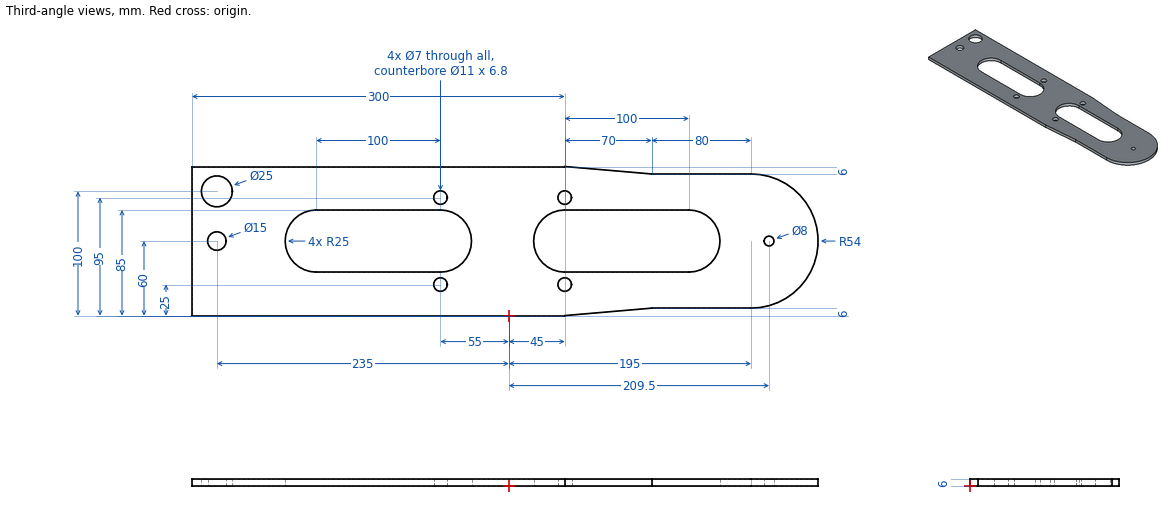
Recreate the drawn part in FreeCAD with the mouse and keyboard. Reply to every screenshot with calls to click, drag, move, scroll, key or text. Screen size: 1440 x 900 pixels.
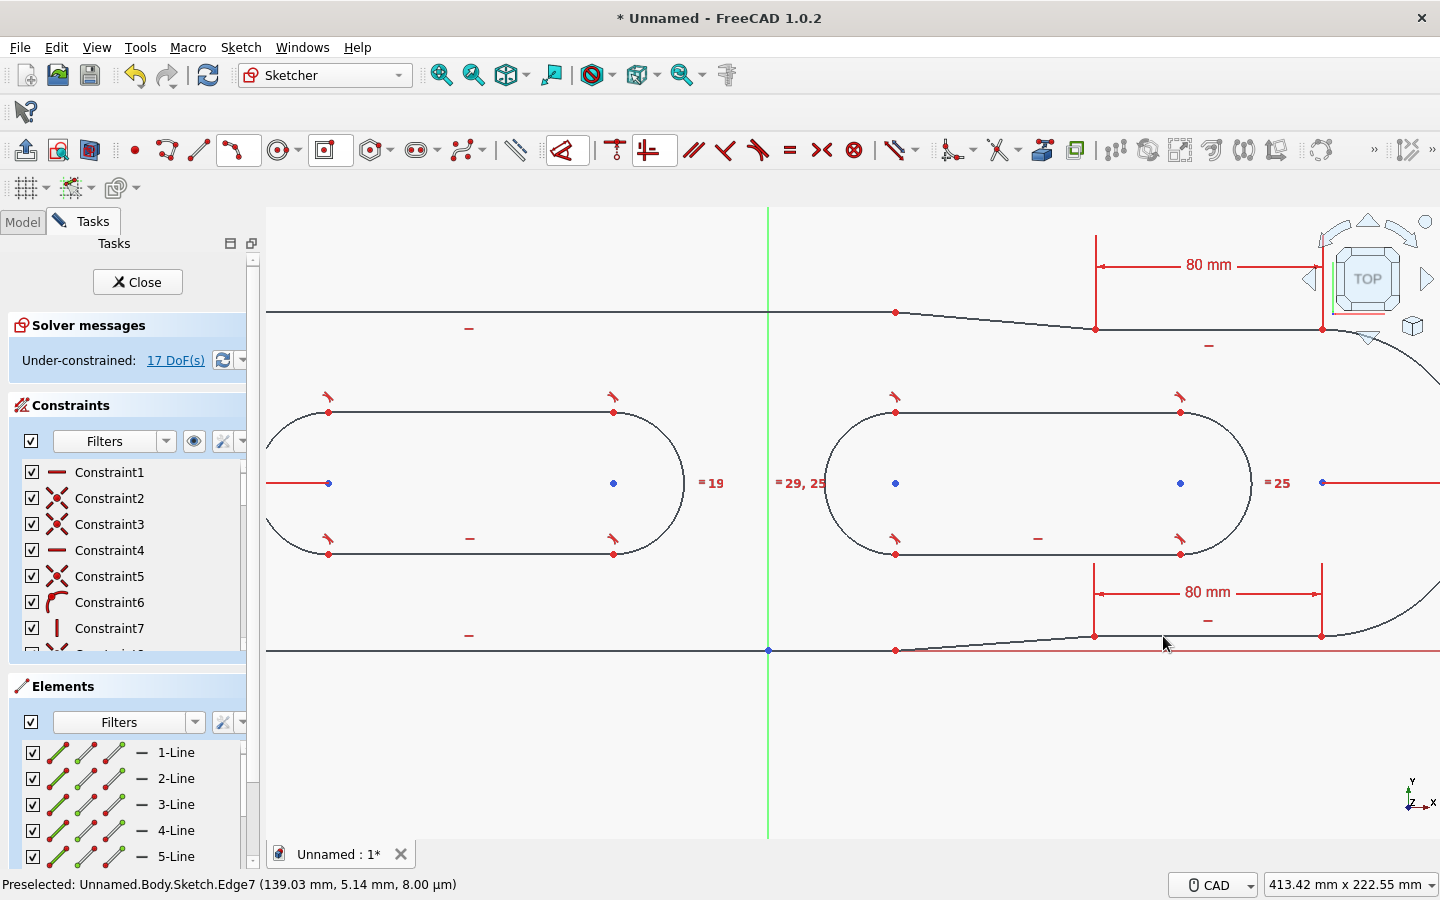
scroll(1094, 636, up, 5)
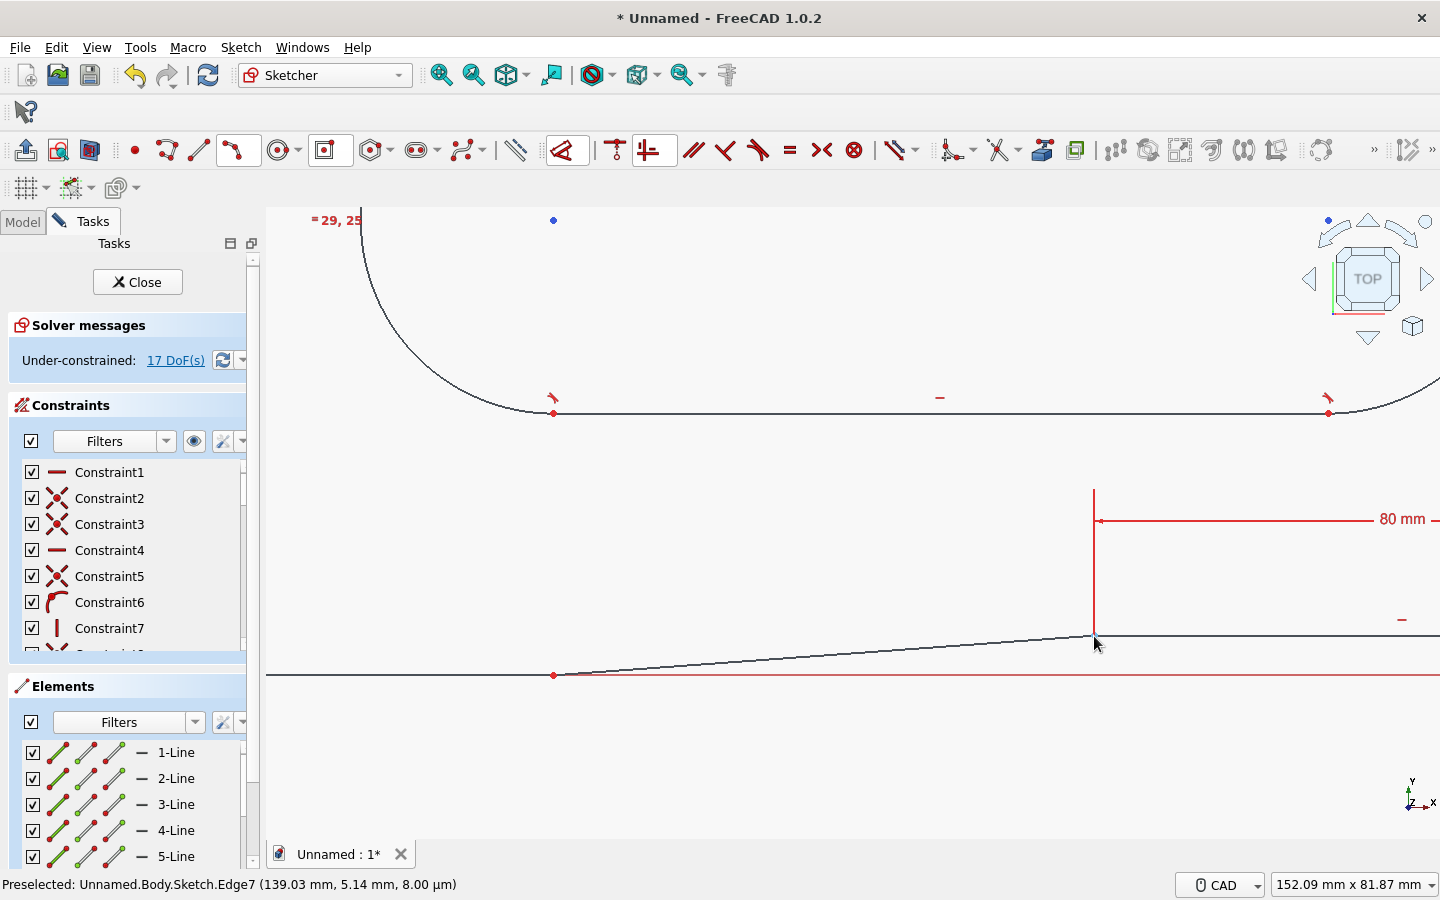
click(1094, 636)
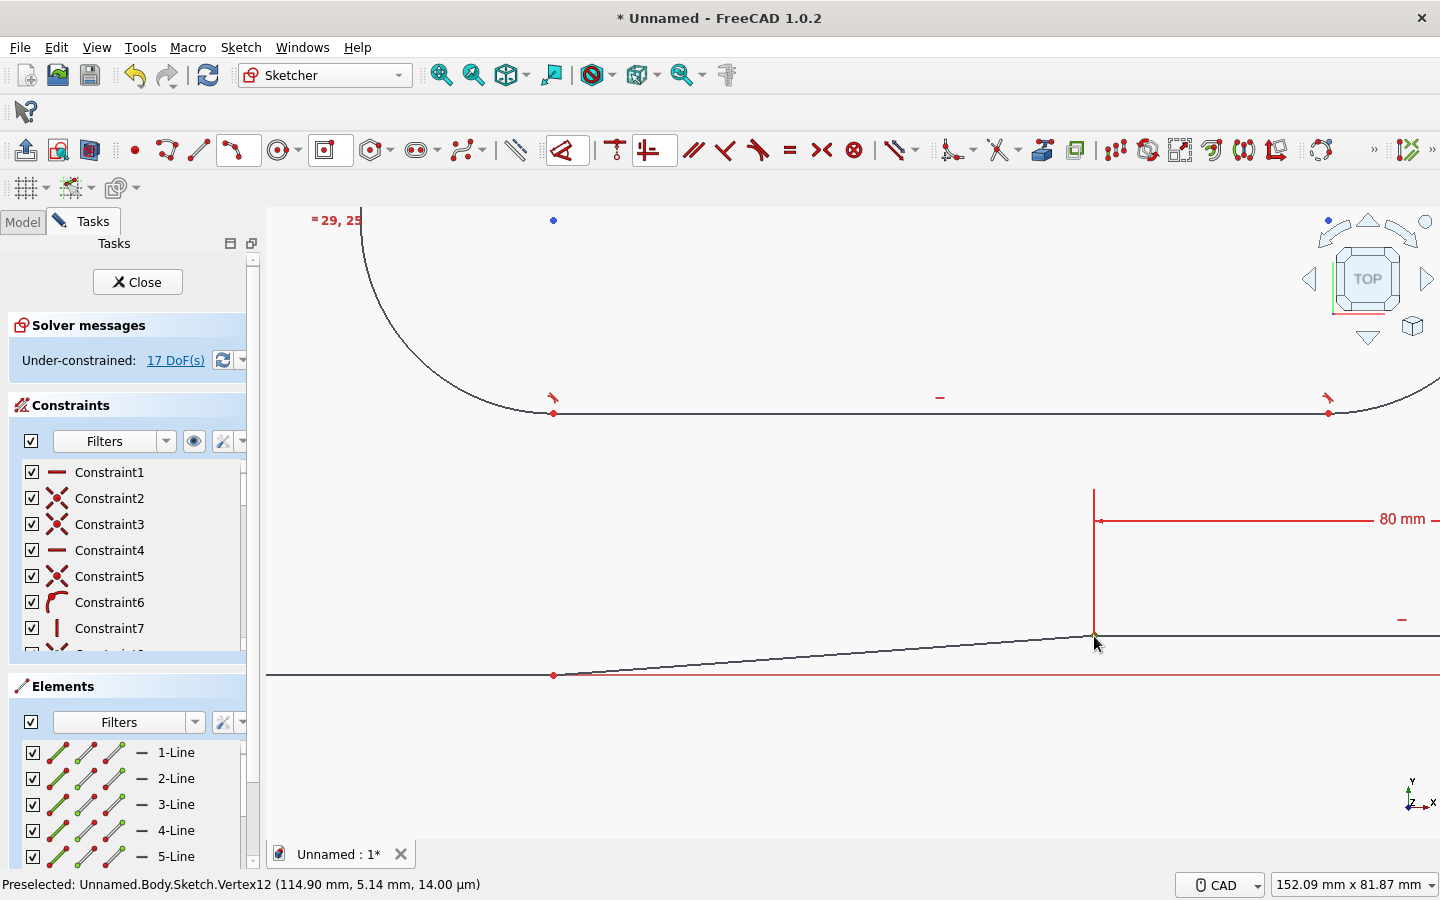
key(i)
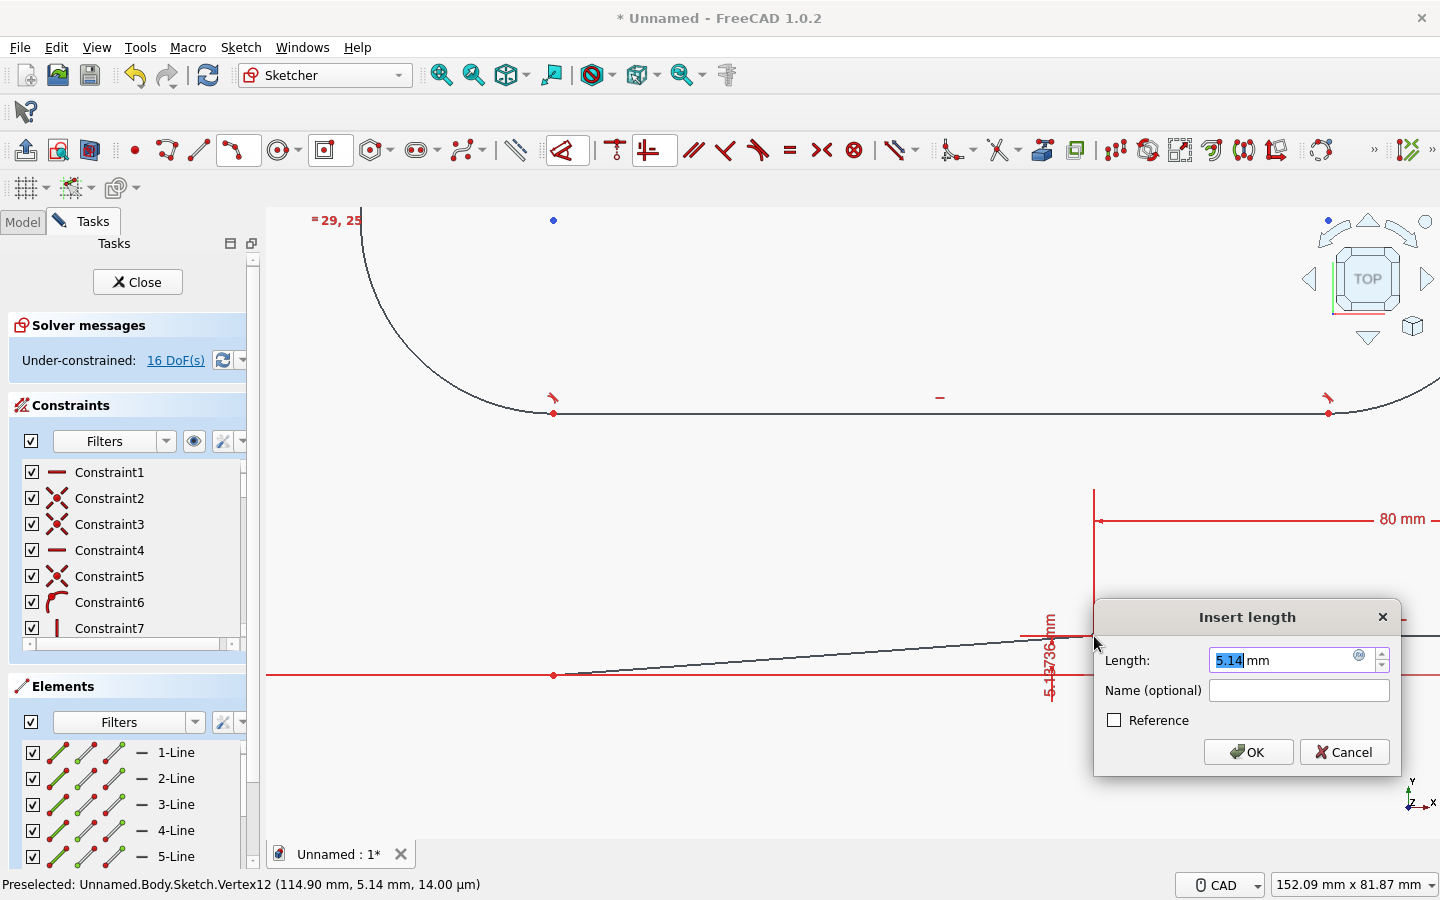
text(6)
key(Return)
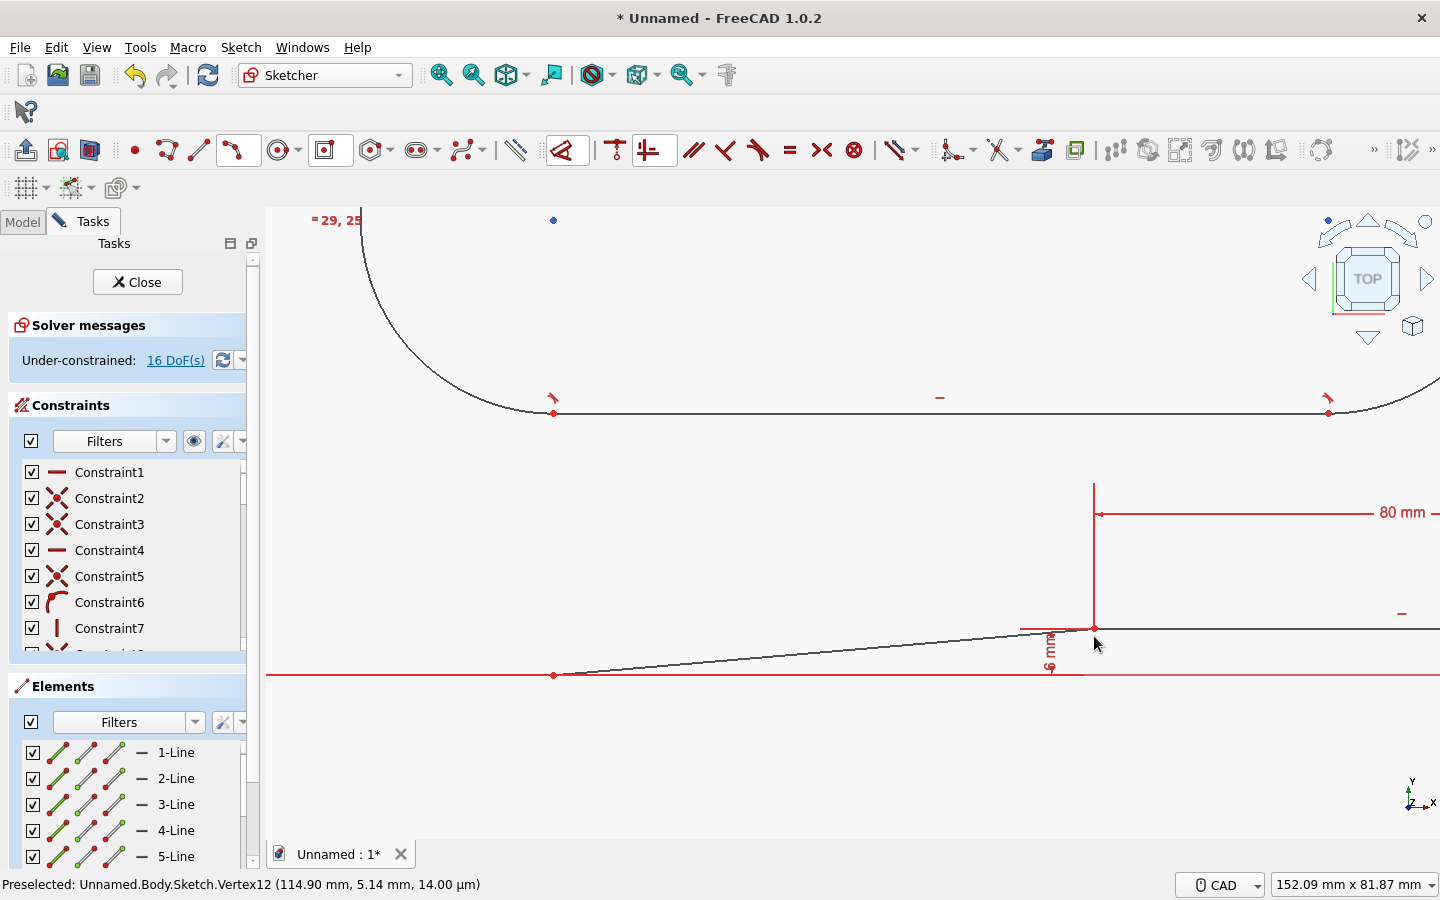
scroll(903, 585, down, 9)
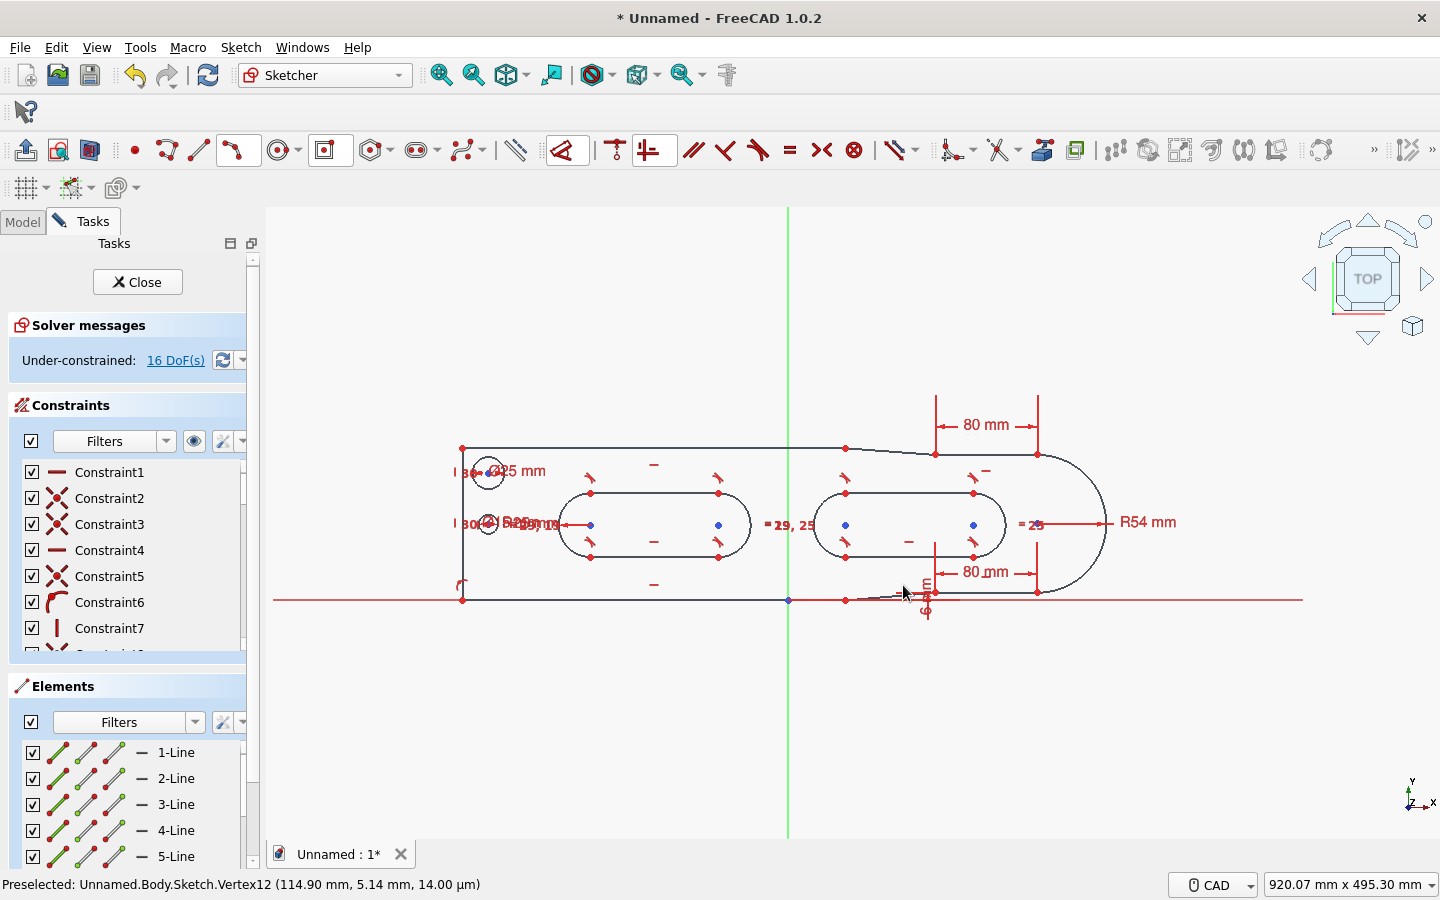
scroll(909, 453, up, 9)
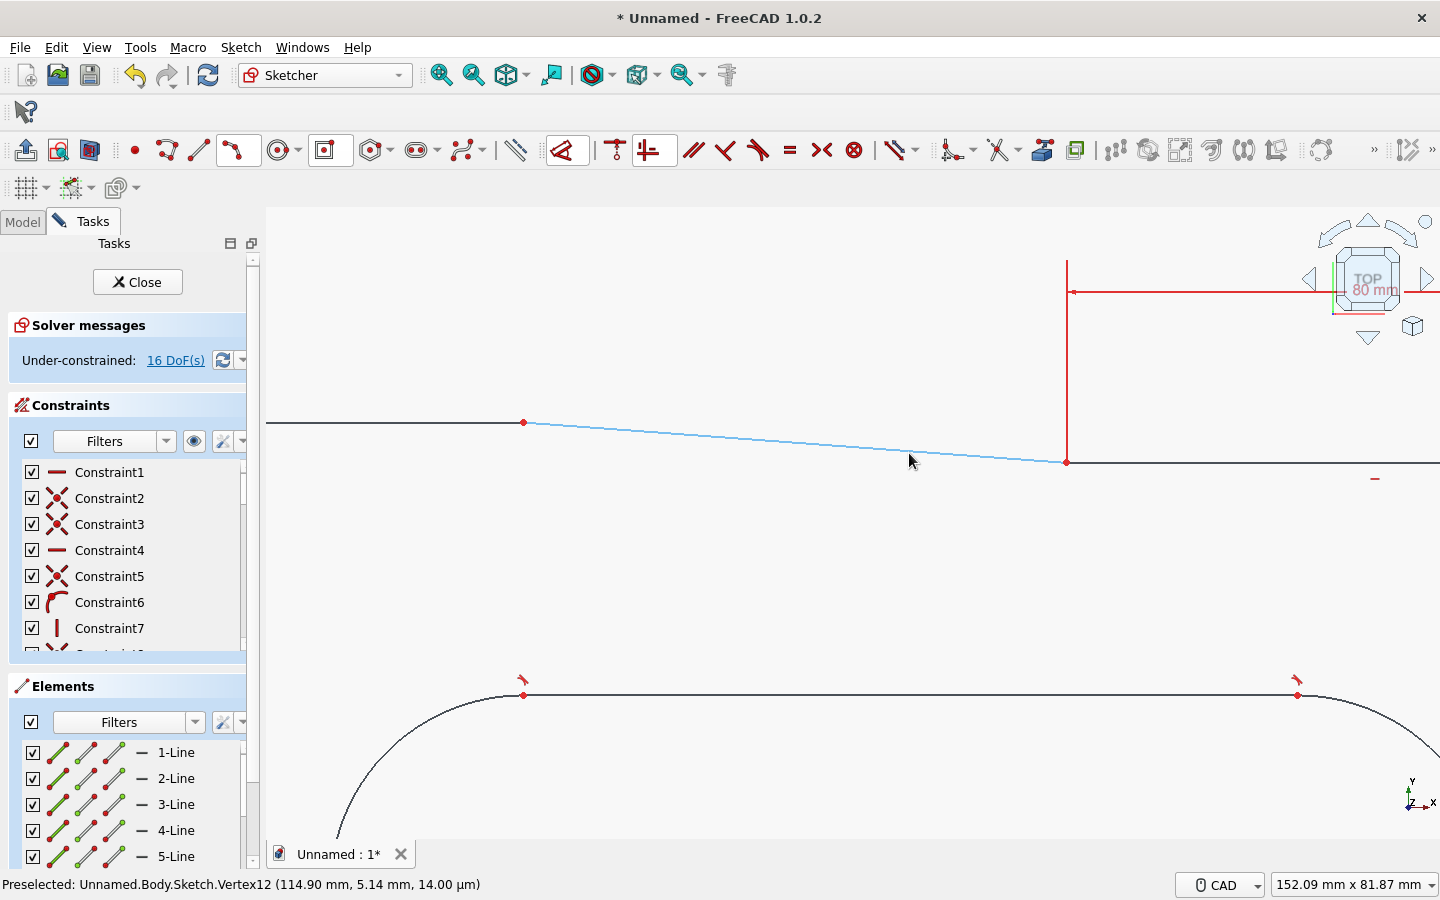
click(904, 451)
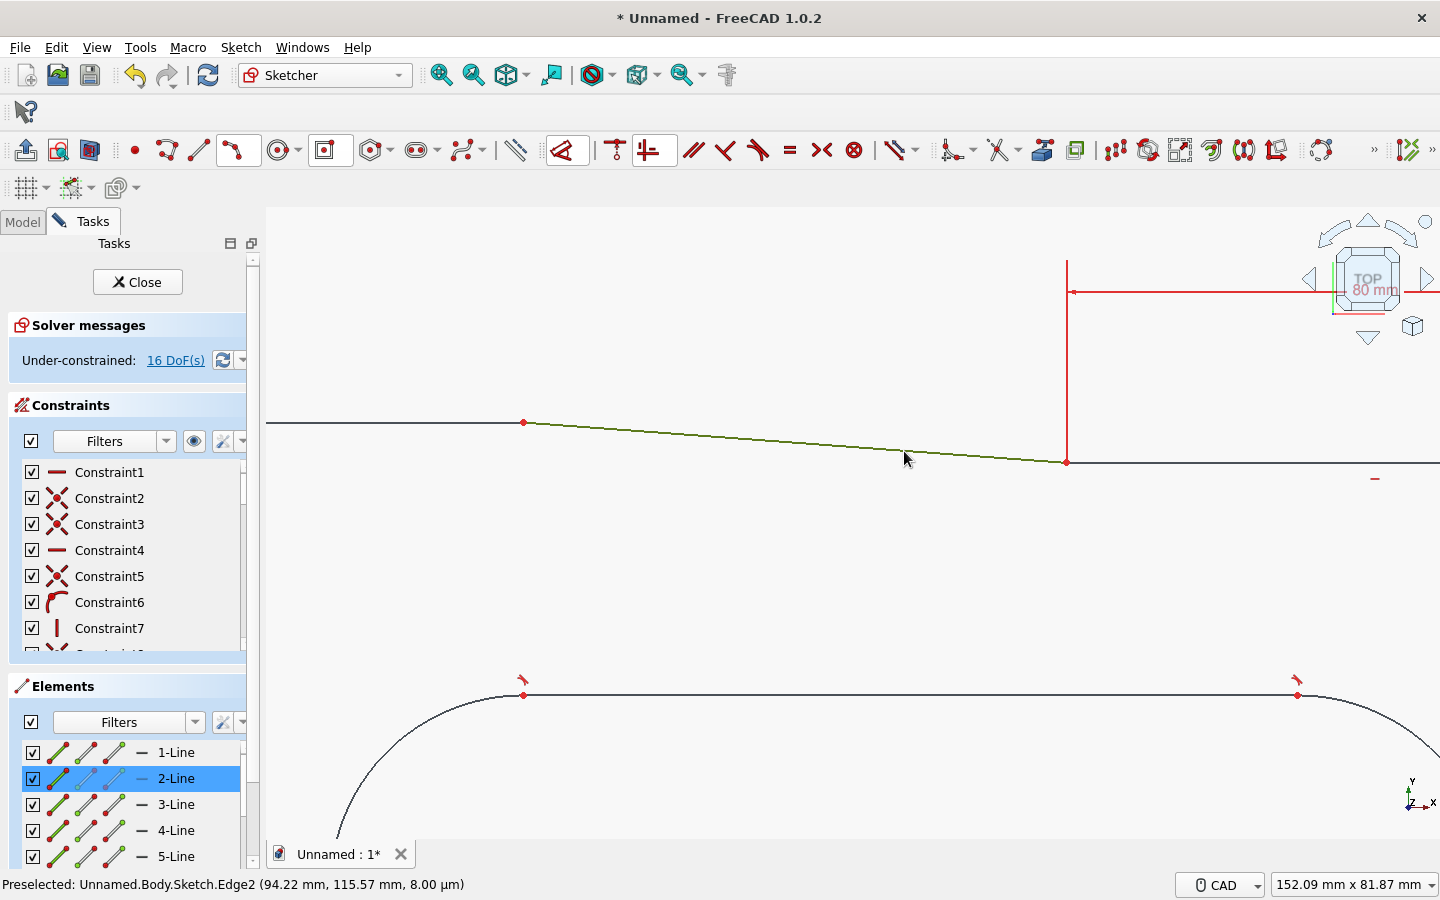
key(i)